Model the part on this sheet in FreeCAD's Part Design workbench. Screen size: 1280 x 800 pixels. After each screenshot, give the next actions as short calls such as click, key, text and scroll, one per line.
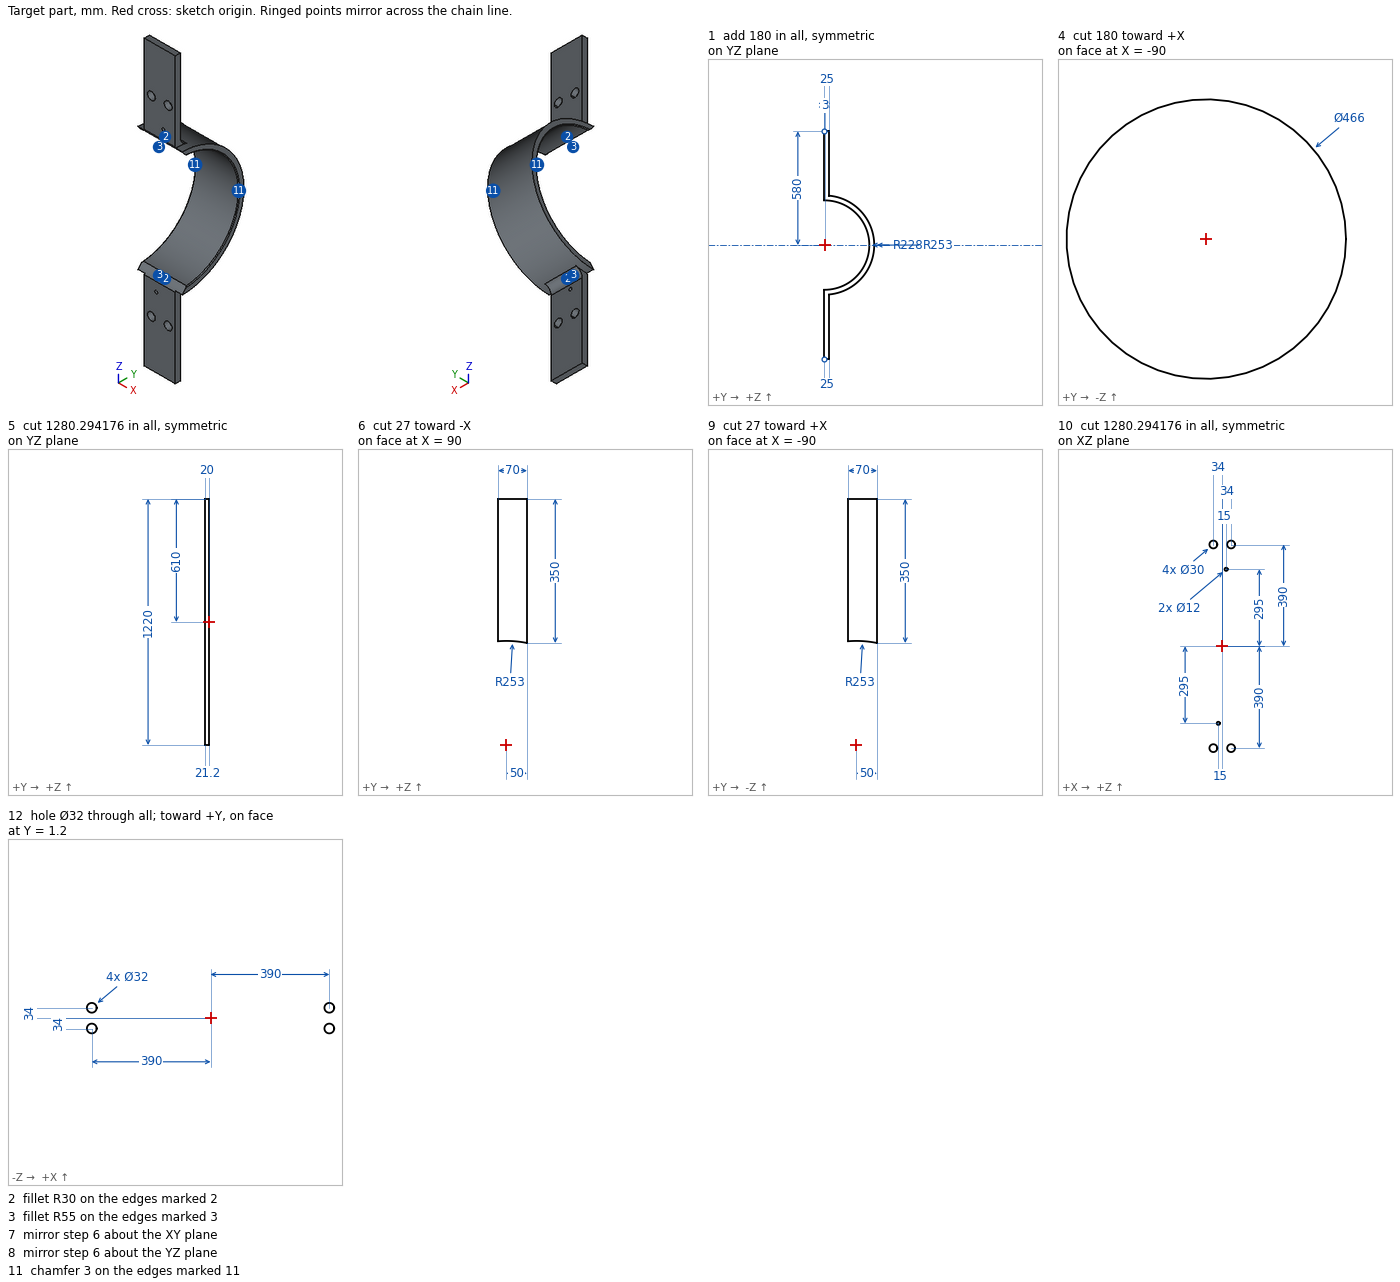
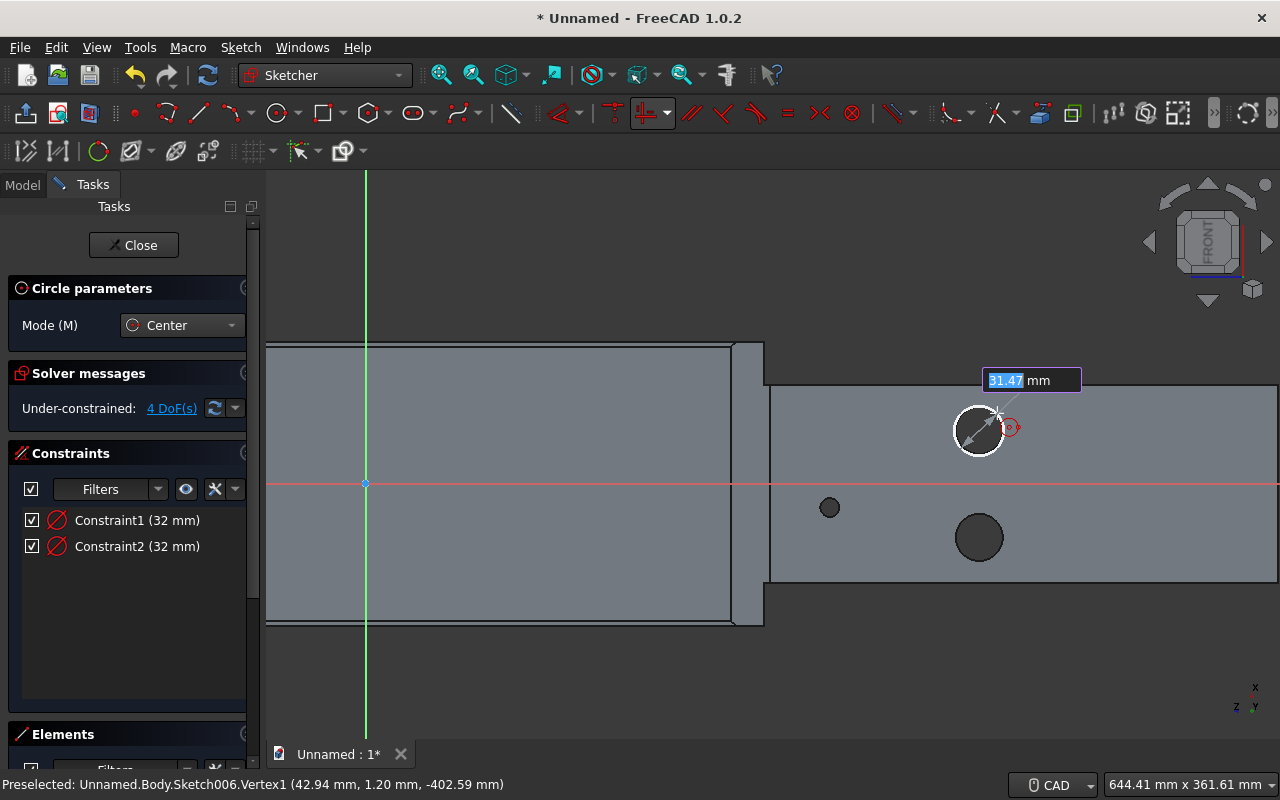
text(32)
key(Return)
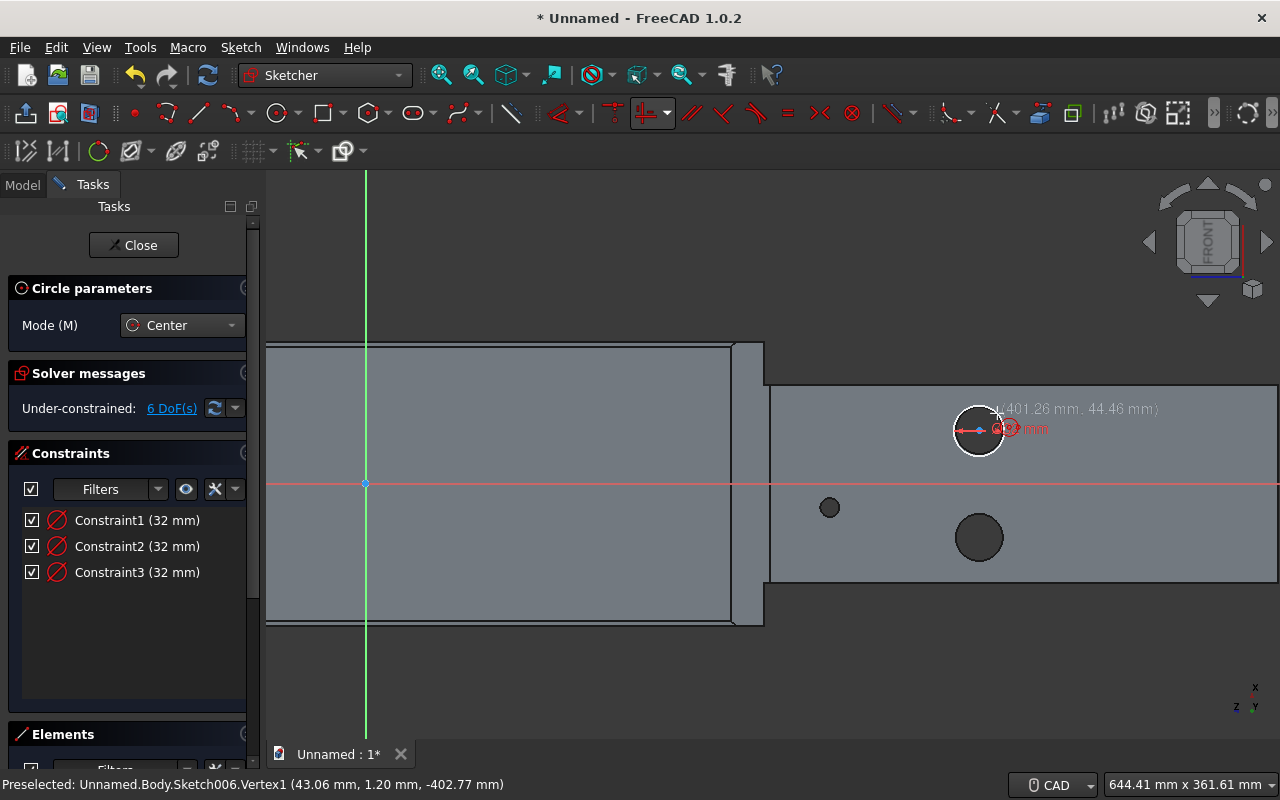
click(979, 537)
move(997, 520)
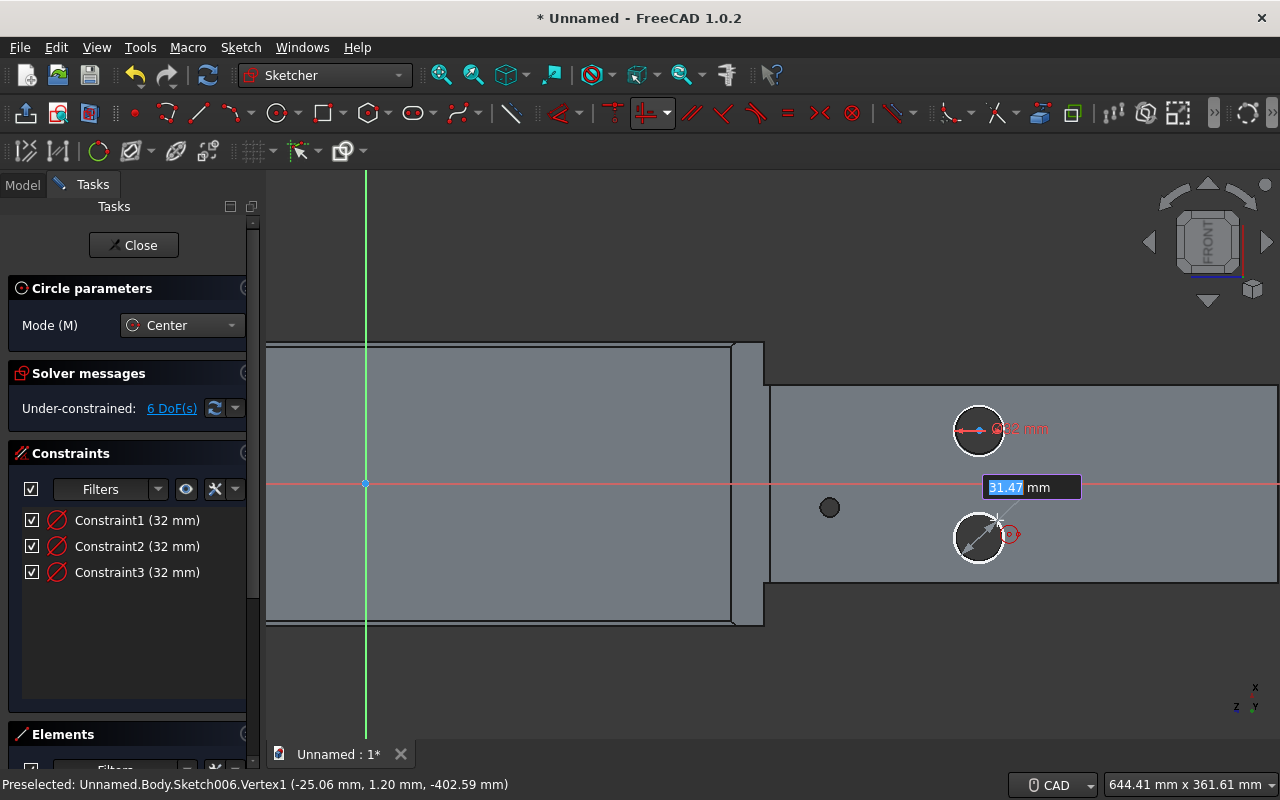
text(32)
key(Return)
key(Escape)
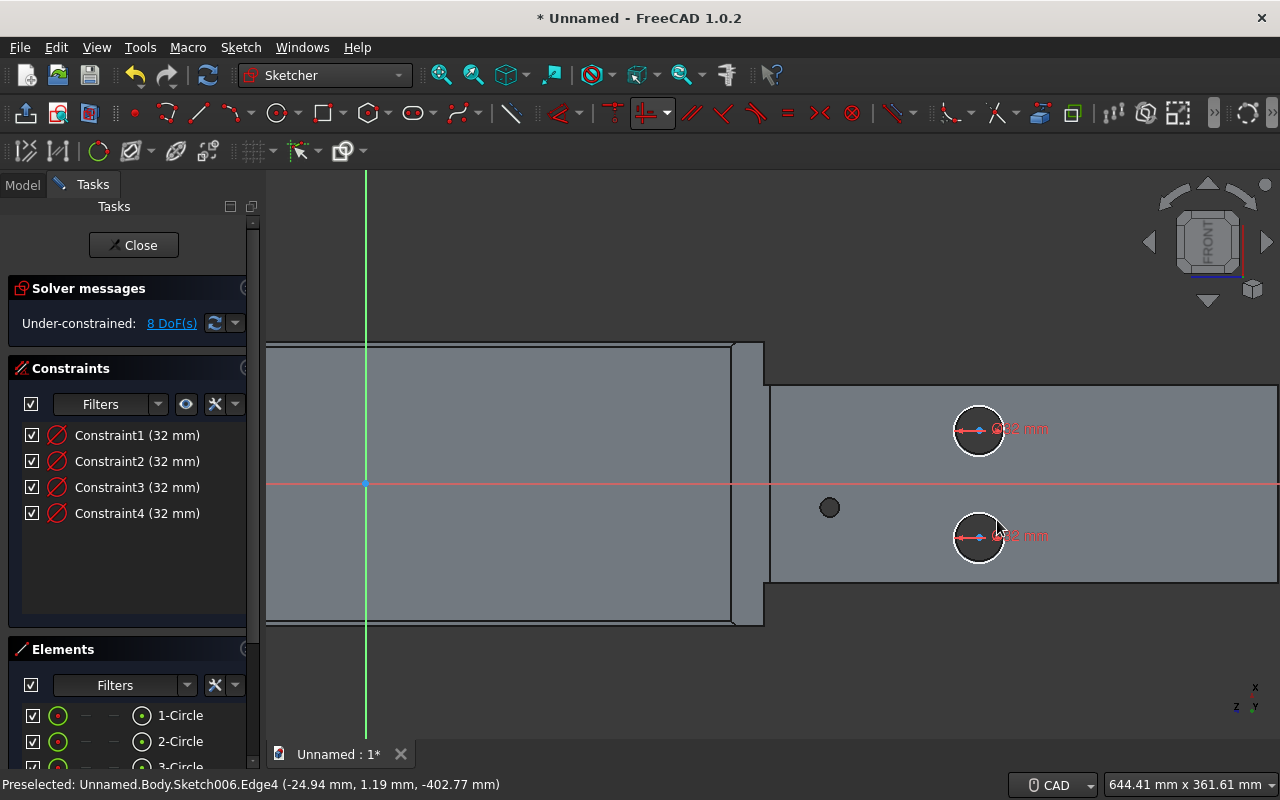
scroll(981, 430, down, 4)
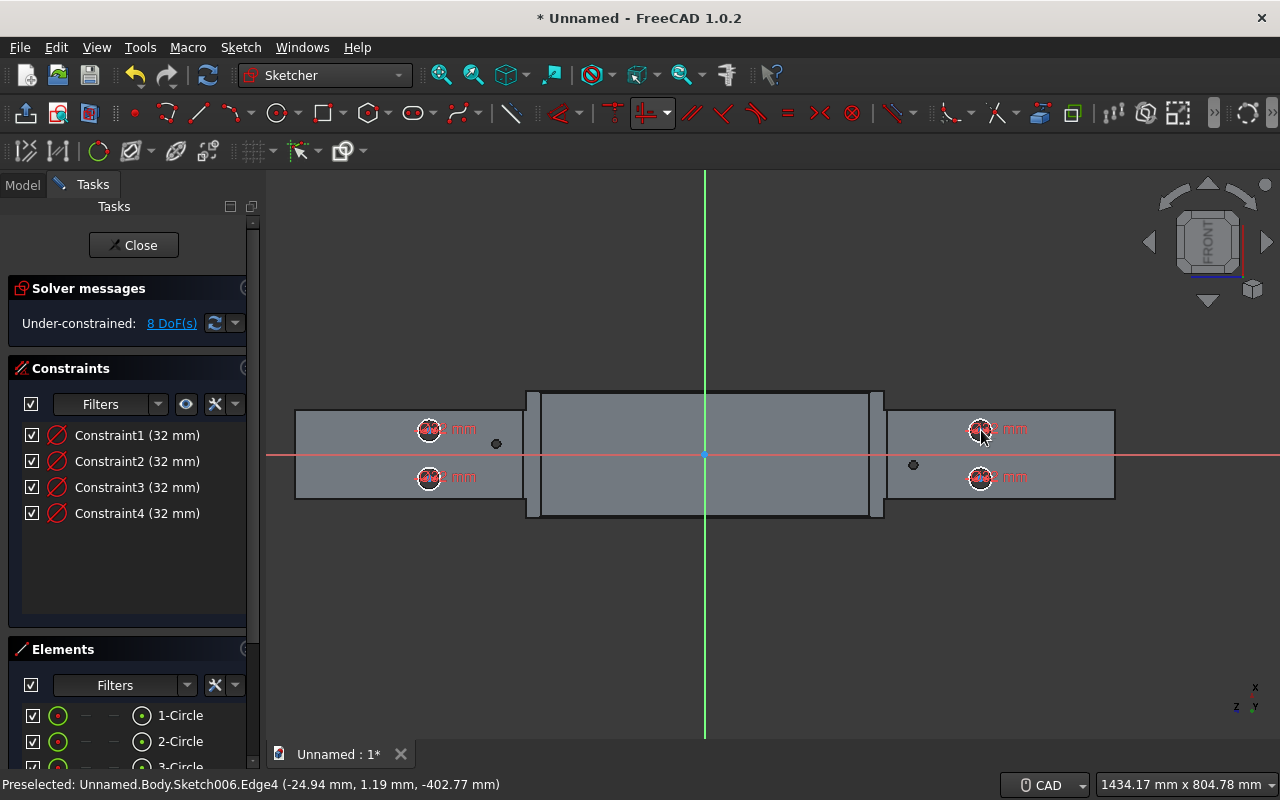
click(429, 479)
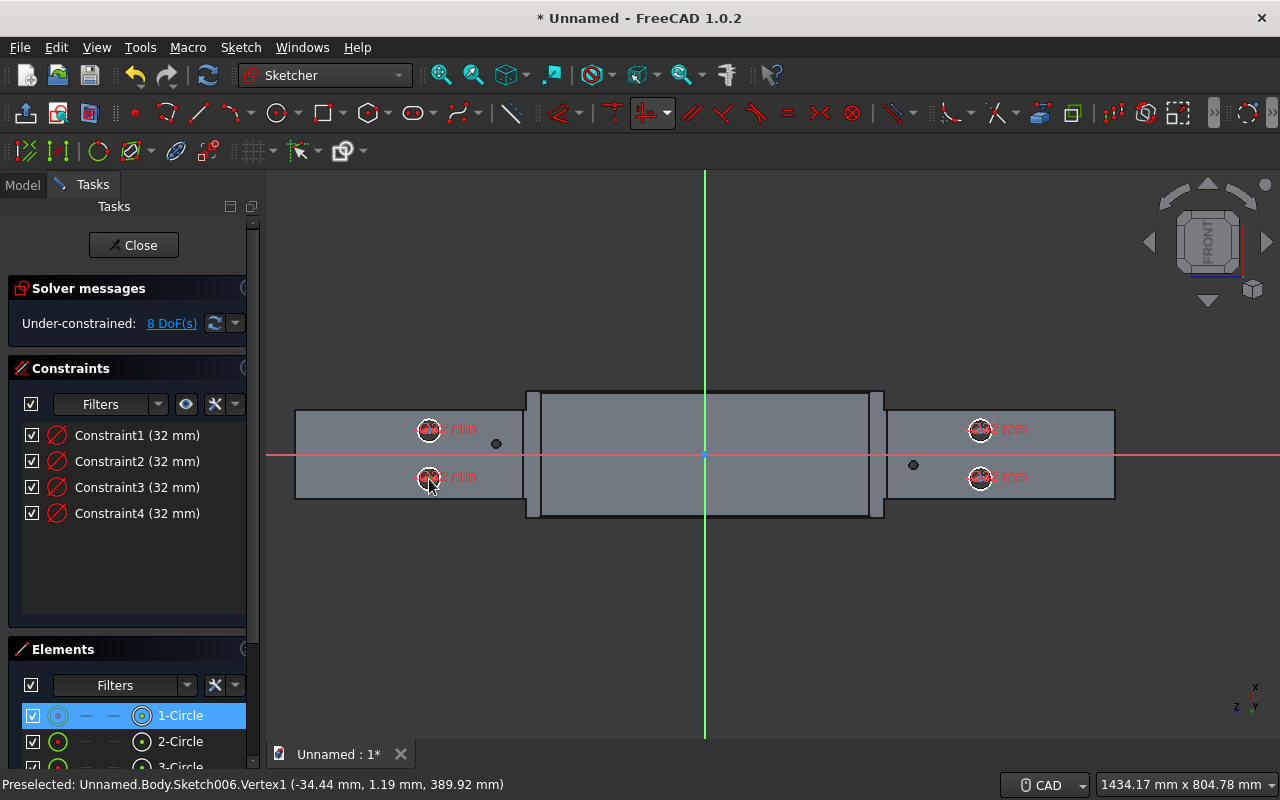
click(429, 431)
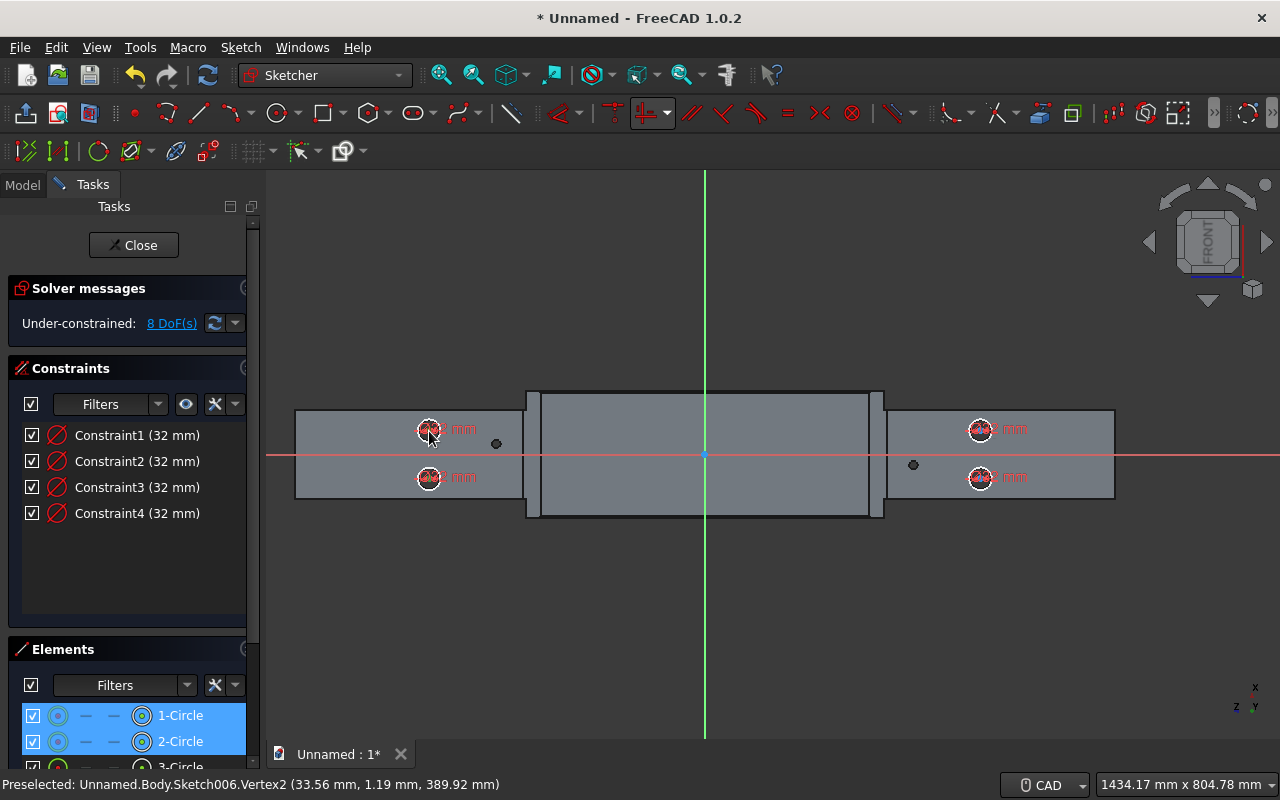
click(670, 114)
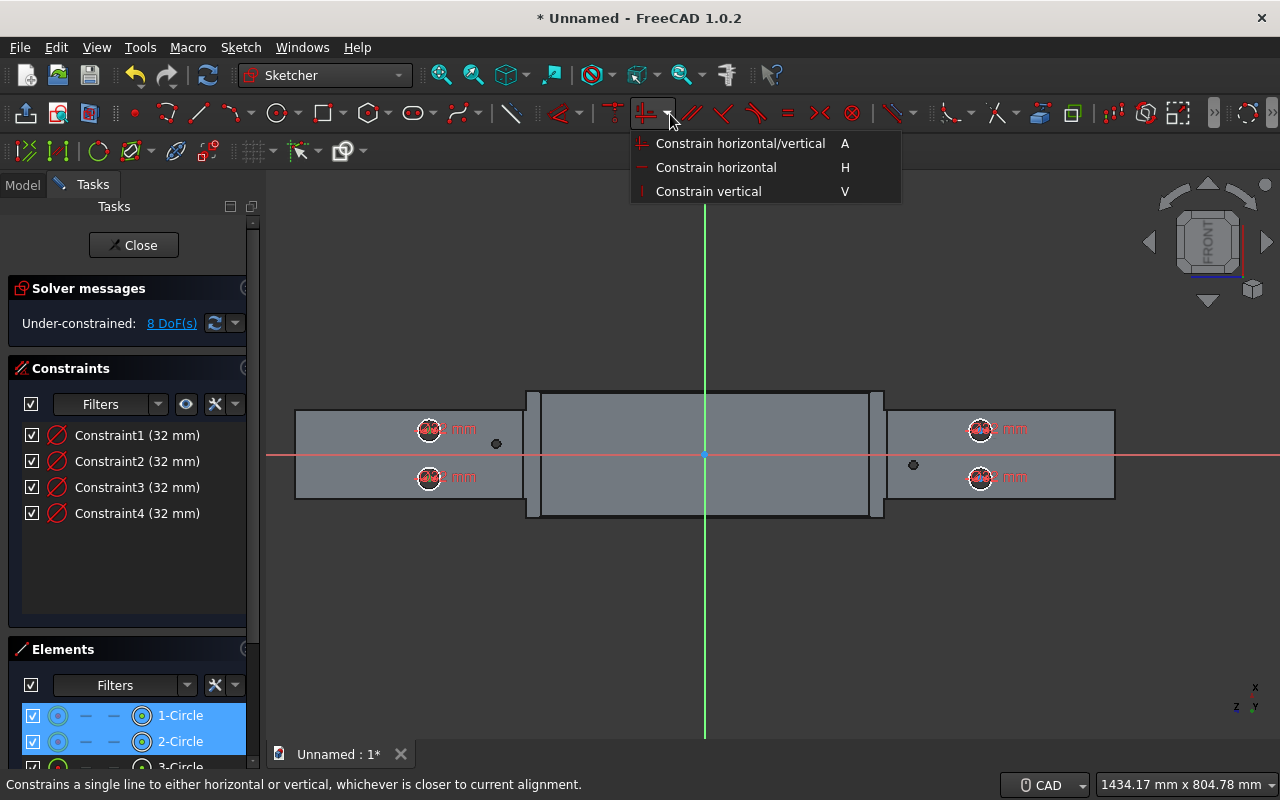
click(766, 191)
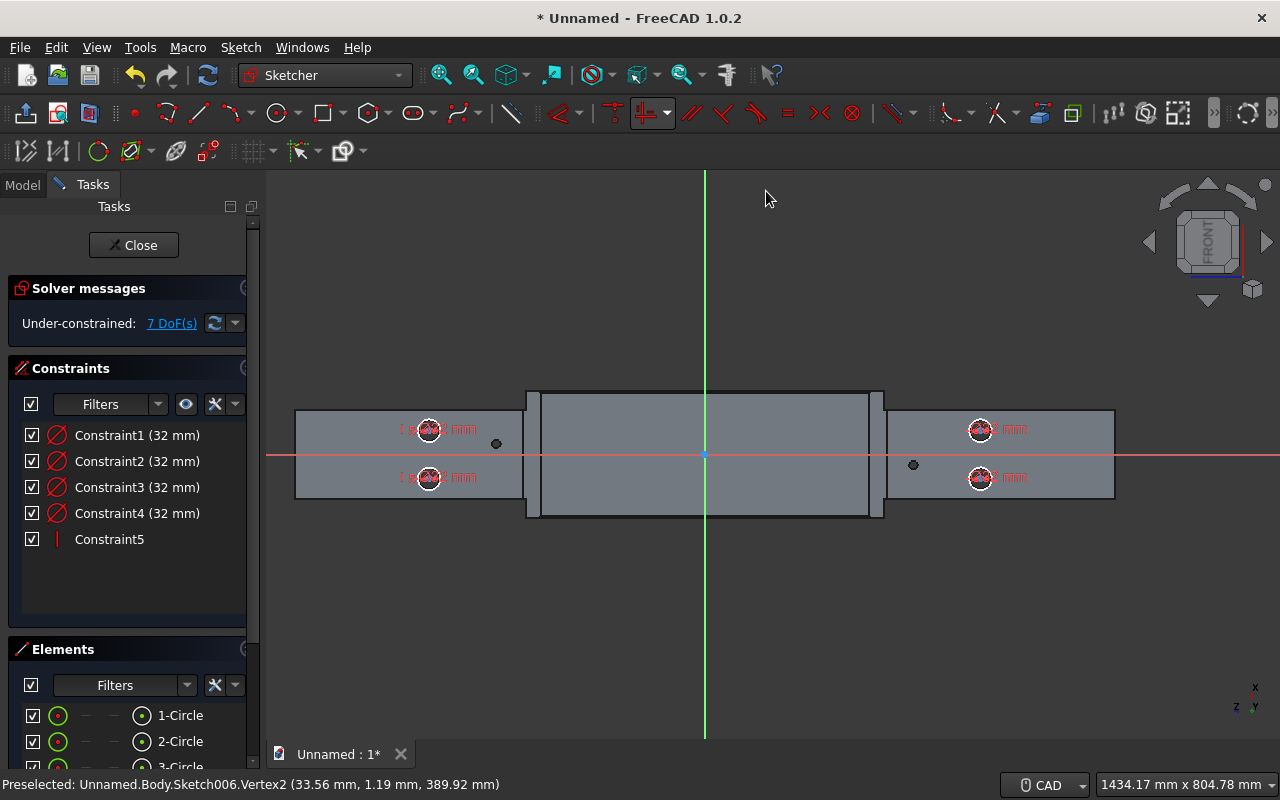
click(429, 431)